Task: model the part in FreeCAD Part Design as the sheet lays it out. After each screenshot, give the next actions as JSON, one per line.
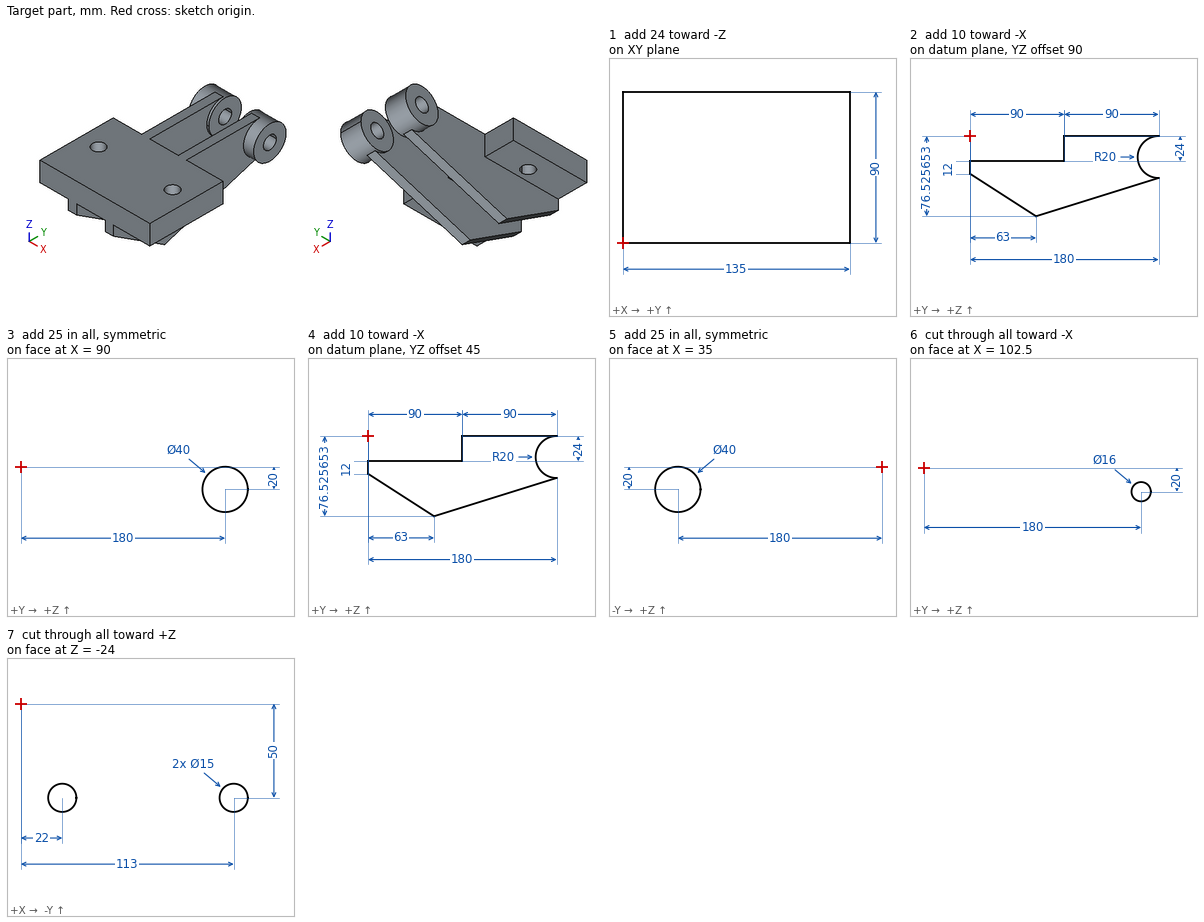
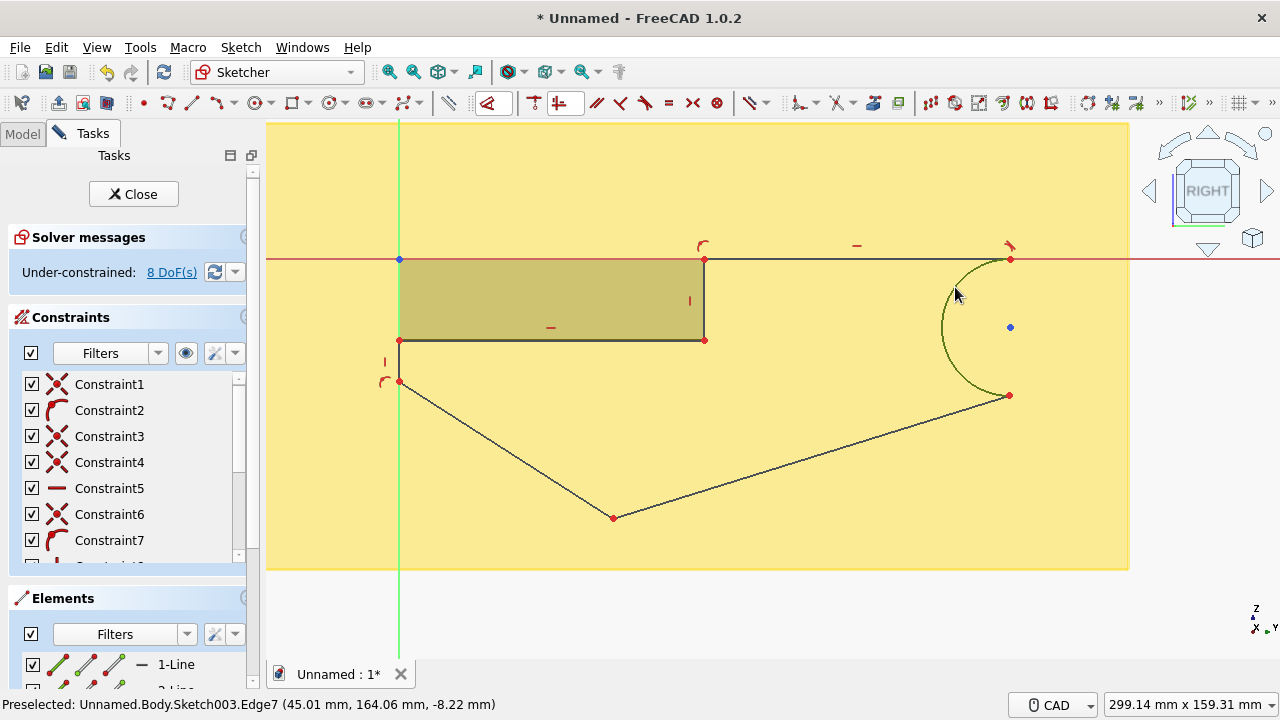
{"action": "left_click", "coordinate": [506, 104]}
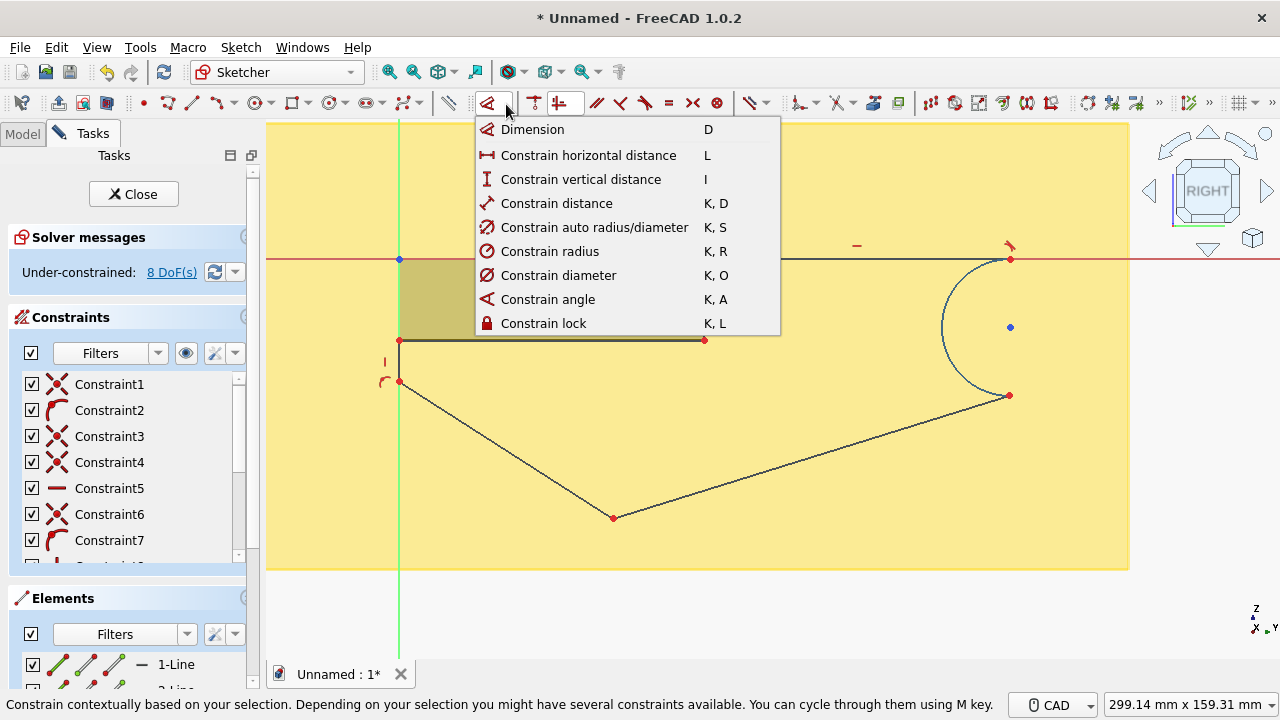
{"action": "left_click", "coordinate": [628, 251]}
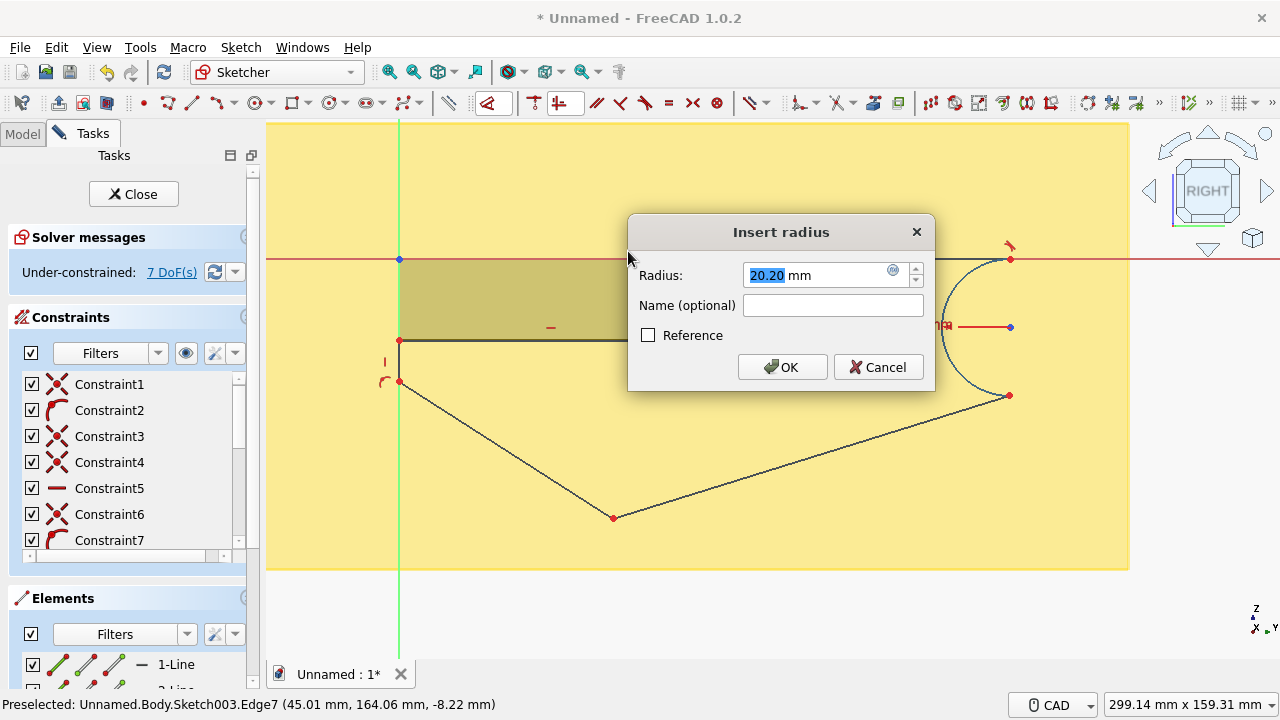
{"action": "type", "text": "20"}
{"action": "key", "text": "Return"}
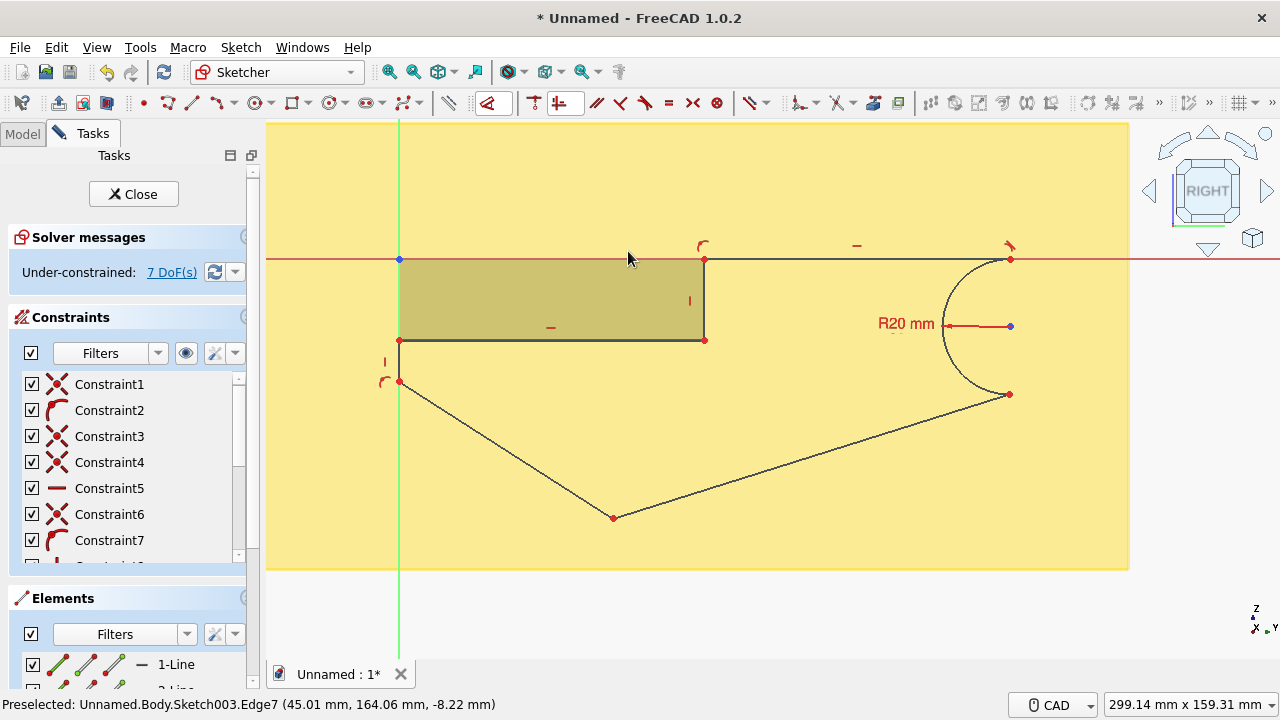
{"action": "left_click", "coordinate": [399, 370]}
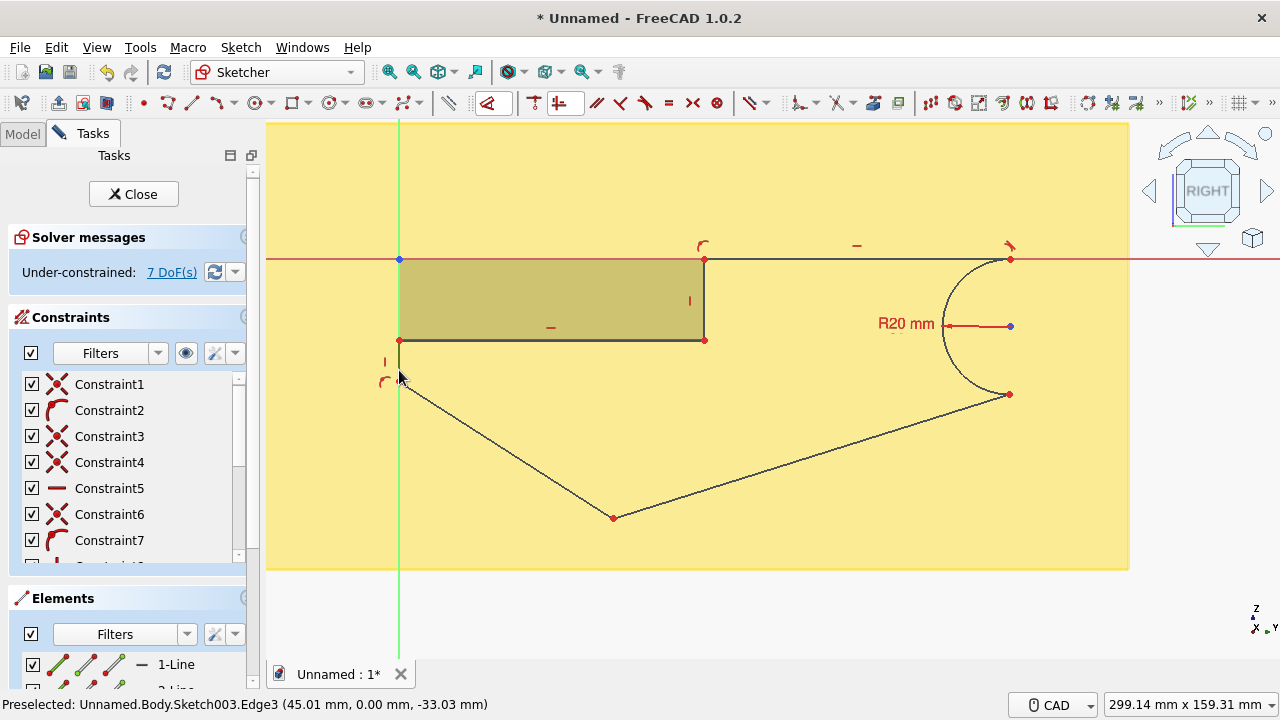
{"action": "key", "text": "i"}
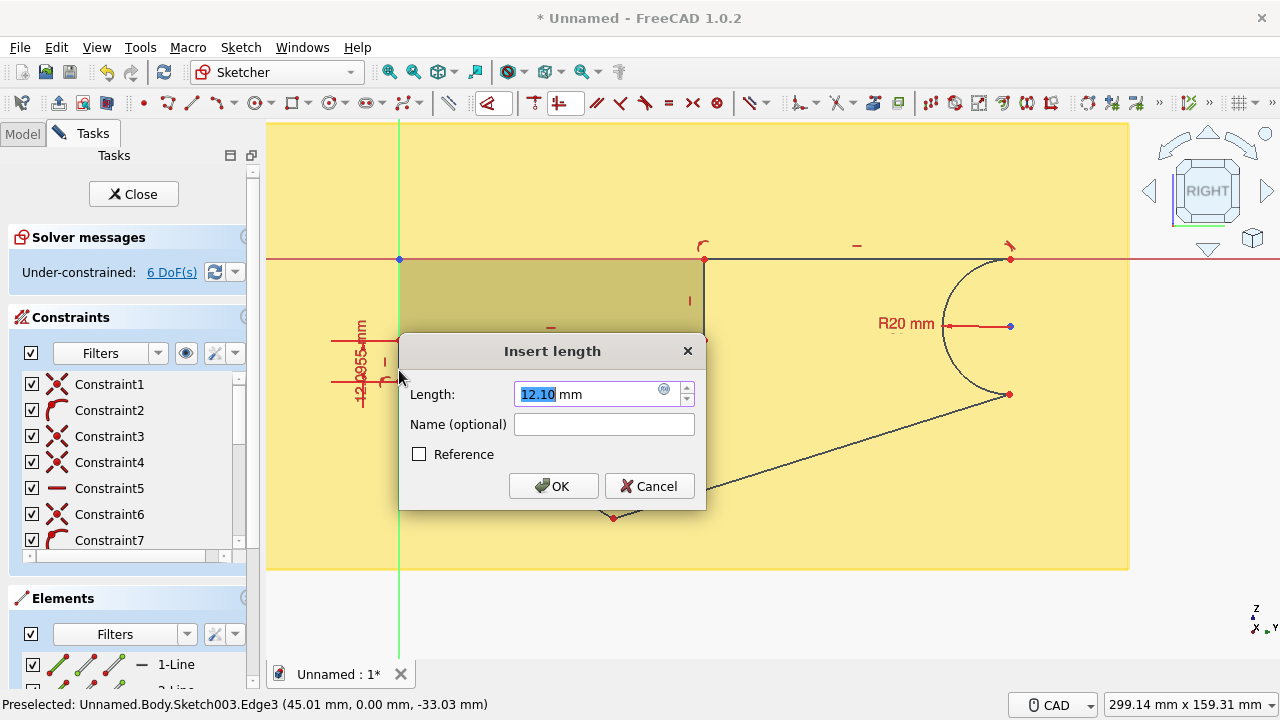
{"action": "type", "text": "12"}
{"action": "key", "text": "Return"}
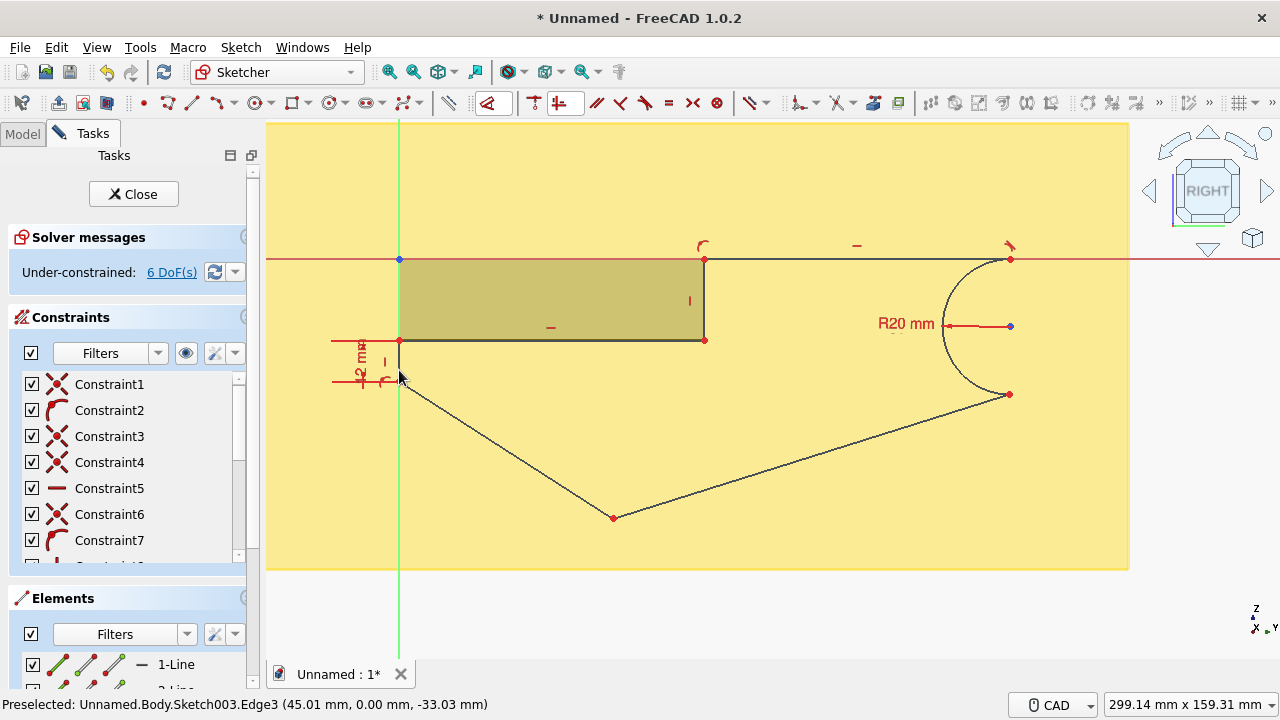
{"action": "left_click", "coordinate": [491, 341]}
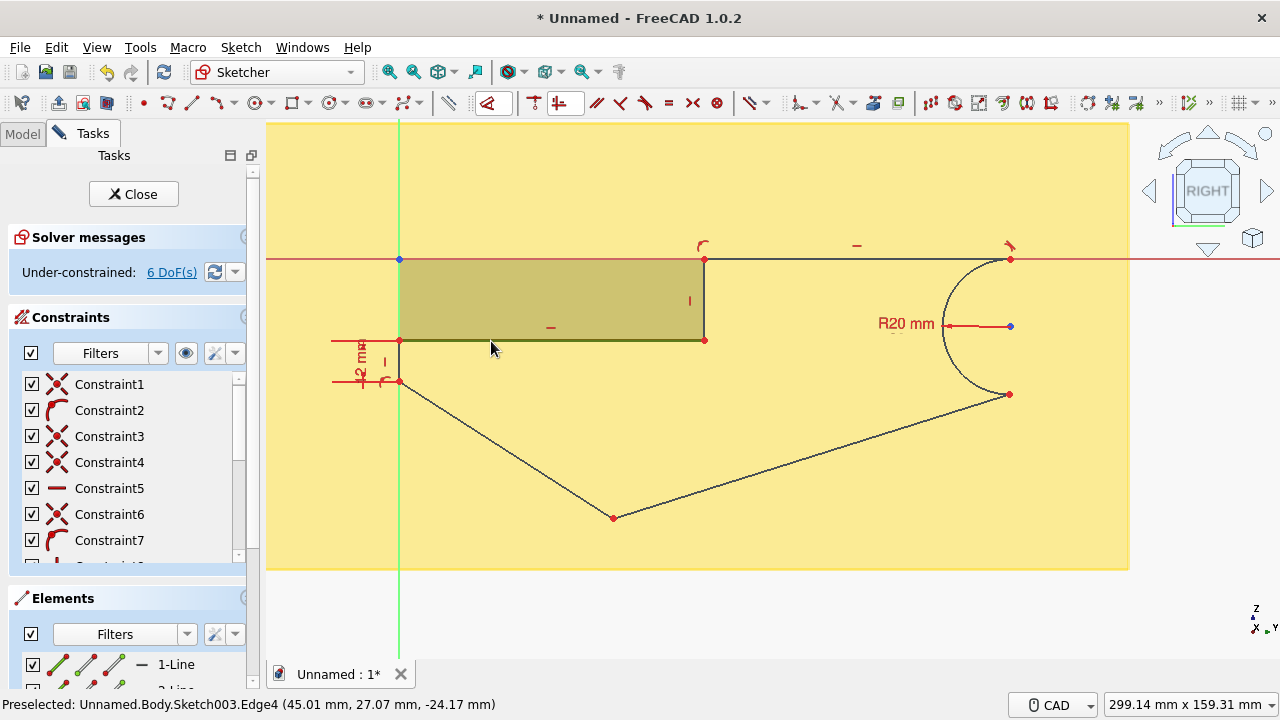
{"action": "left_click", "coordinate": [506, 104]}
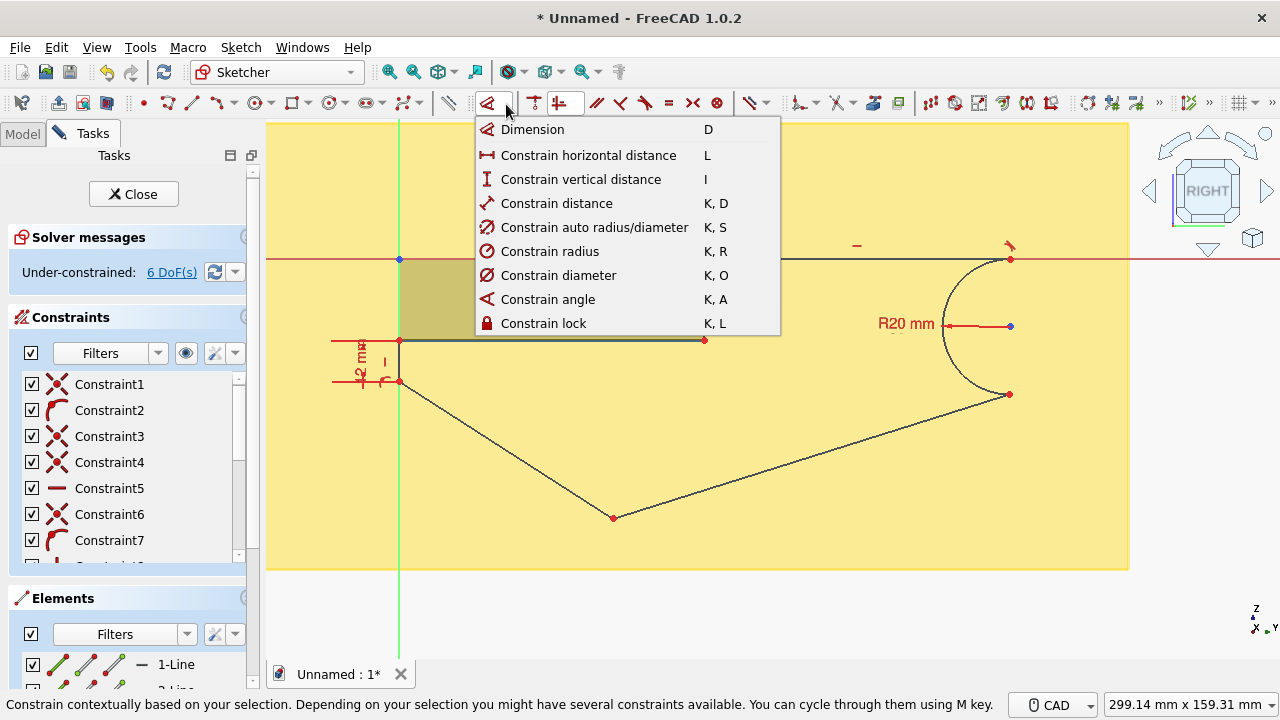
{"action": "left_click", "coordinate": [628, 155]}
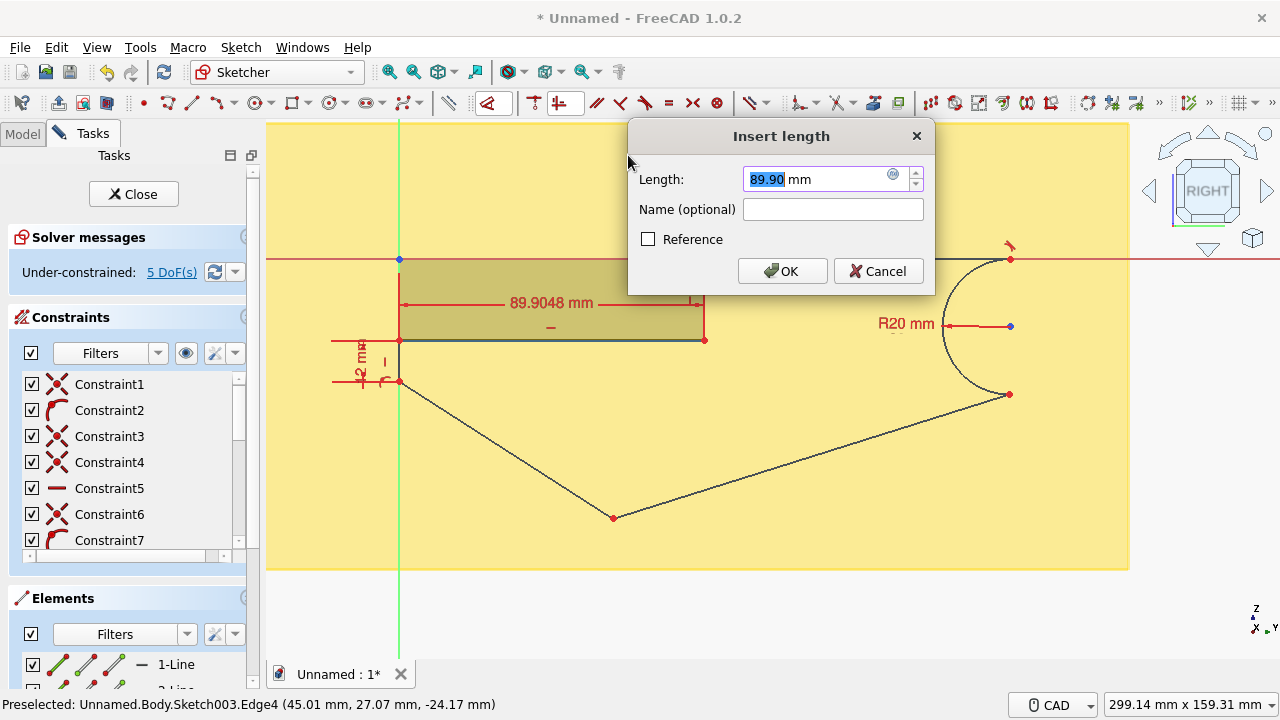
{"action": "type", "text": "90"}
{"action": "key", "text": "Return"}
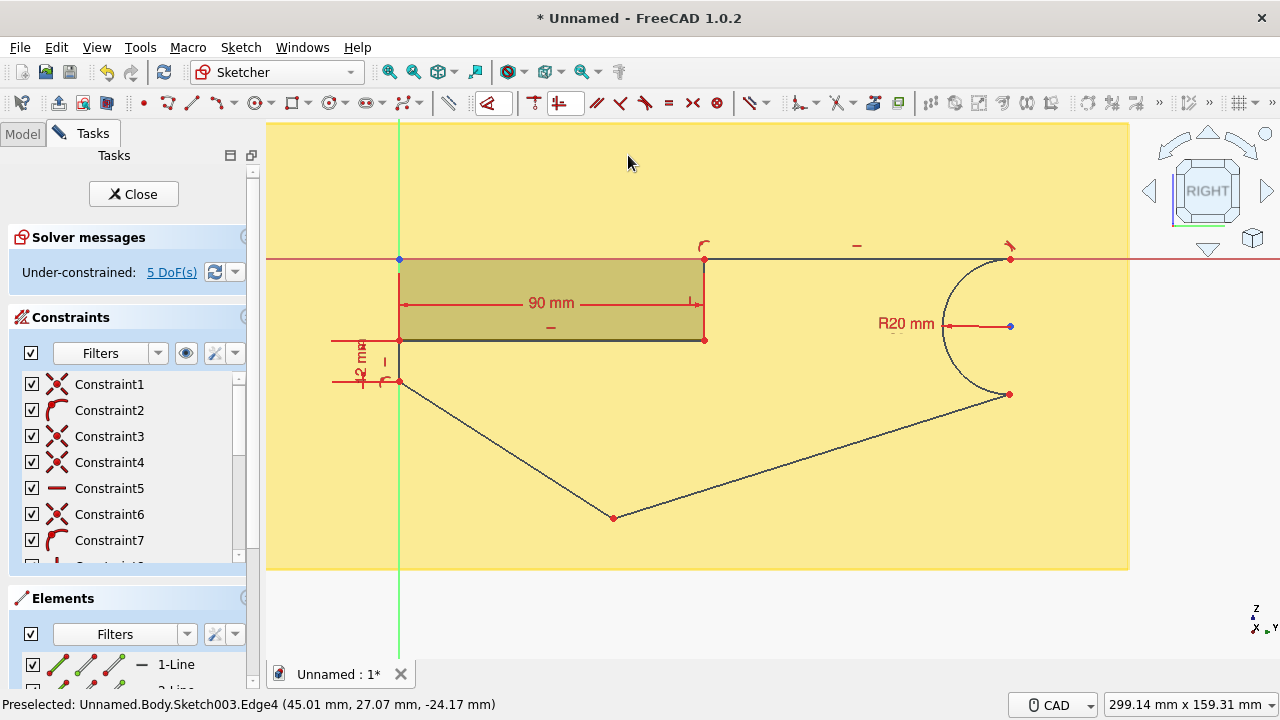
{"action": "left_click", "coordinate": [704, 316]}